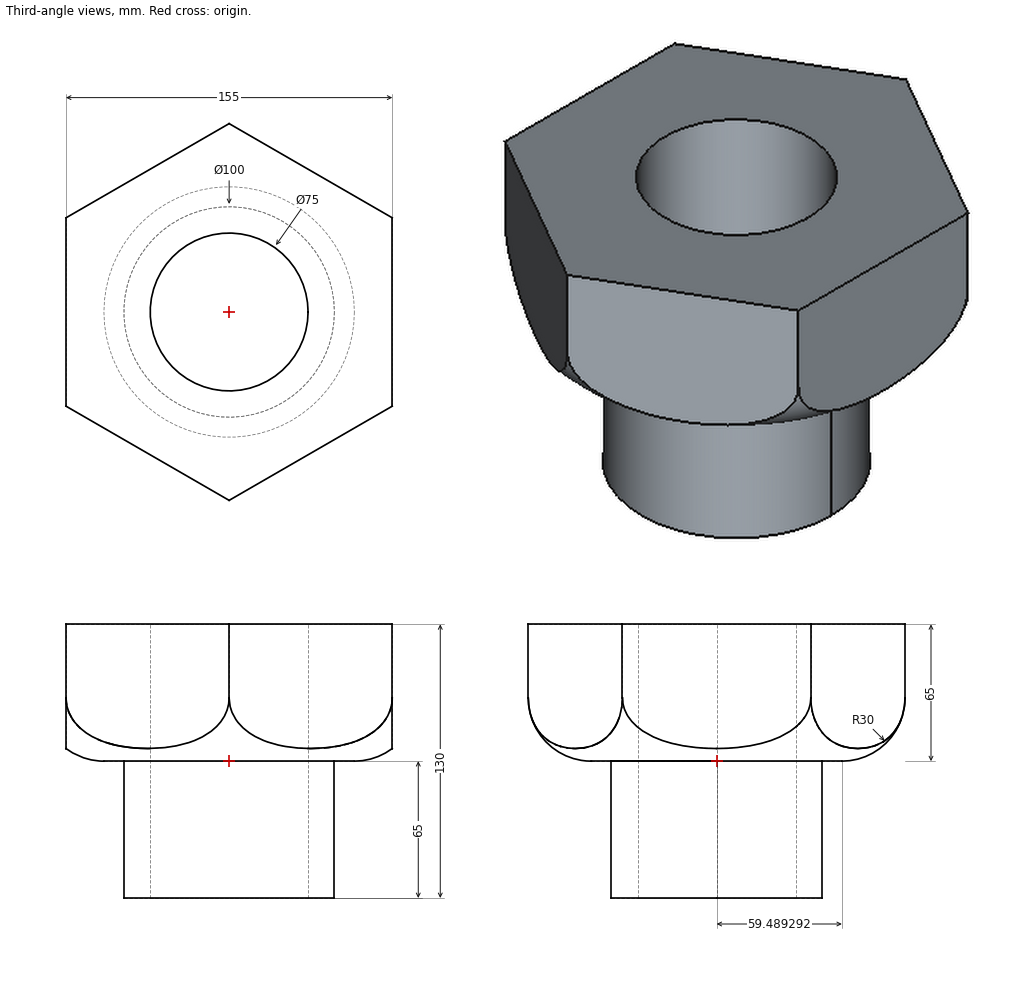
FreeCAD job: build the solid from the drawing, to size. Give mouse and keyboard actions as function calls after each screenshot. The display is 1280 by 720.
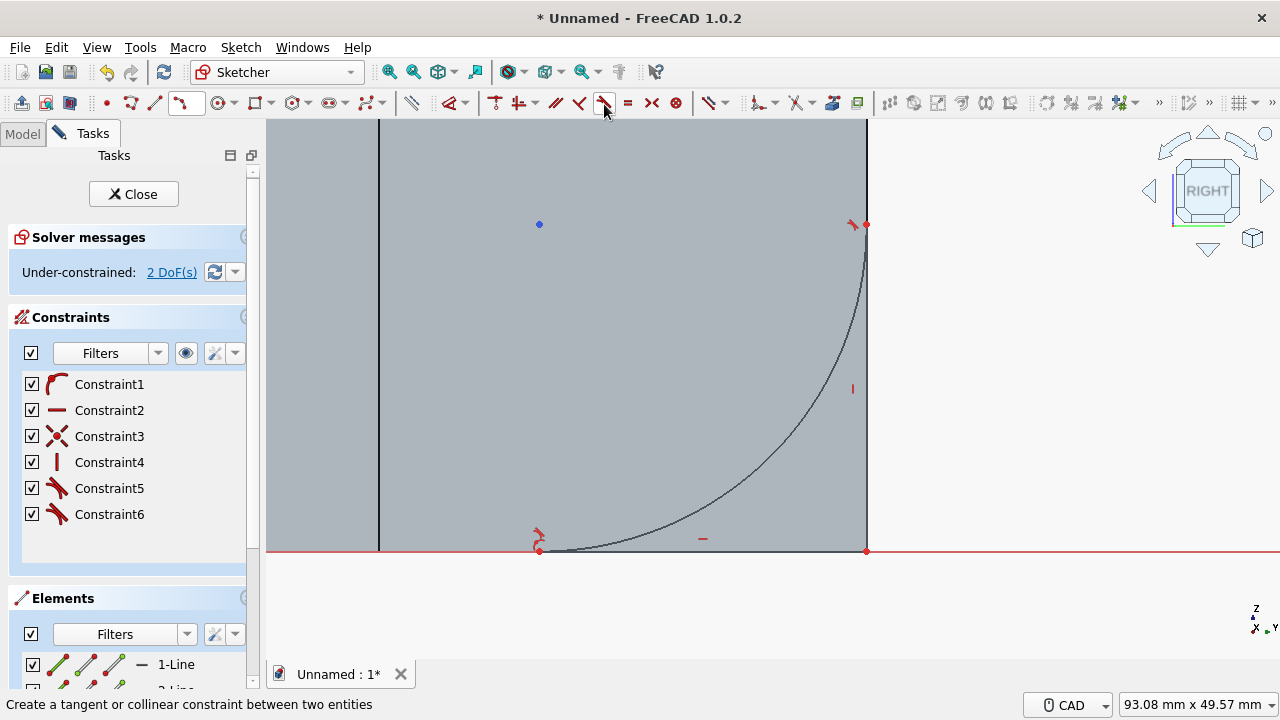
click(688, 516)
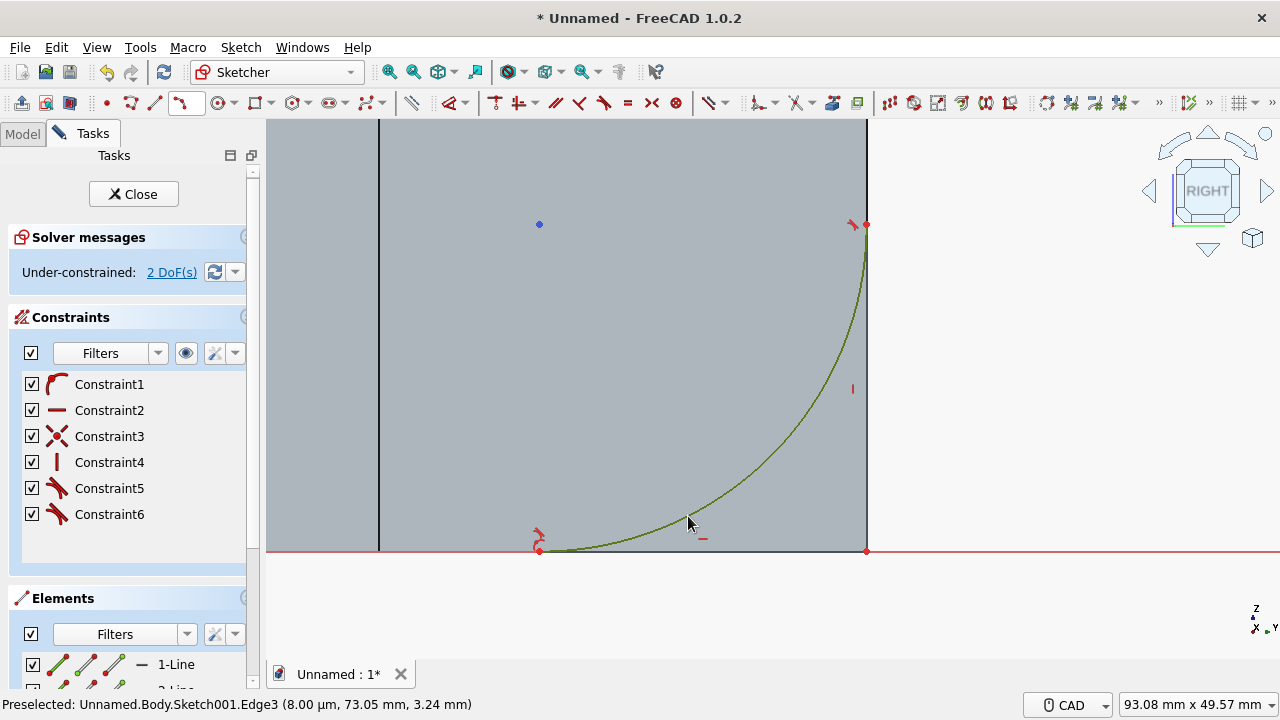
key(k)
key(r)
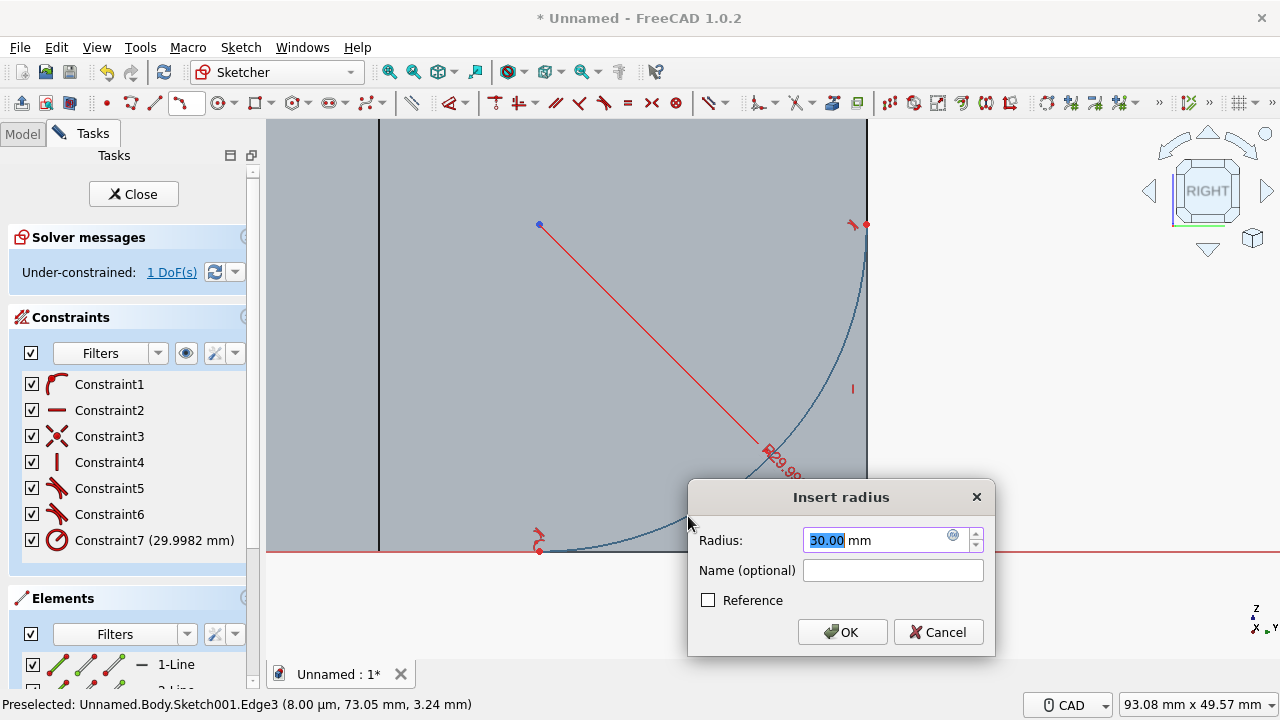
text(30)
key(Return)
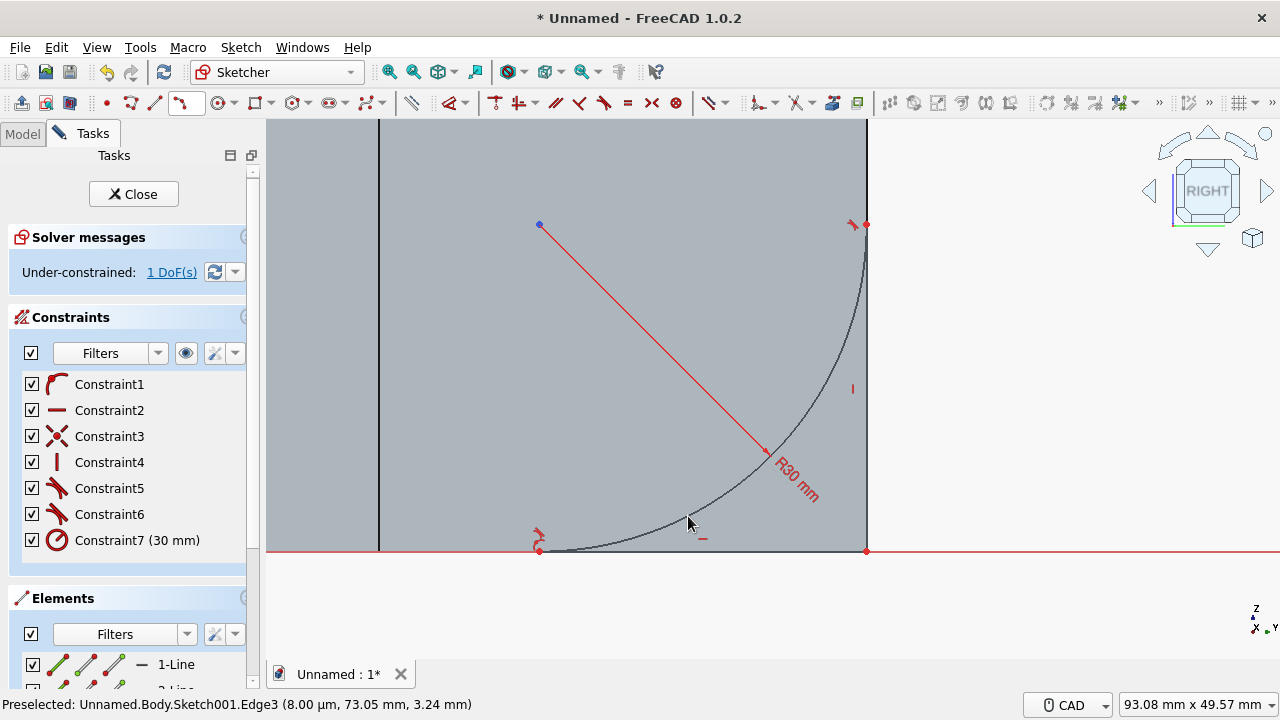
click(540, 552)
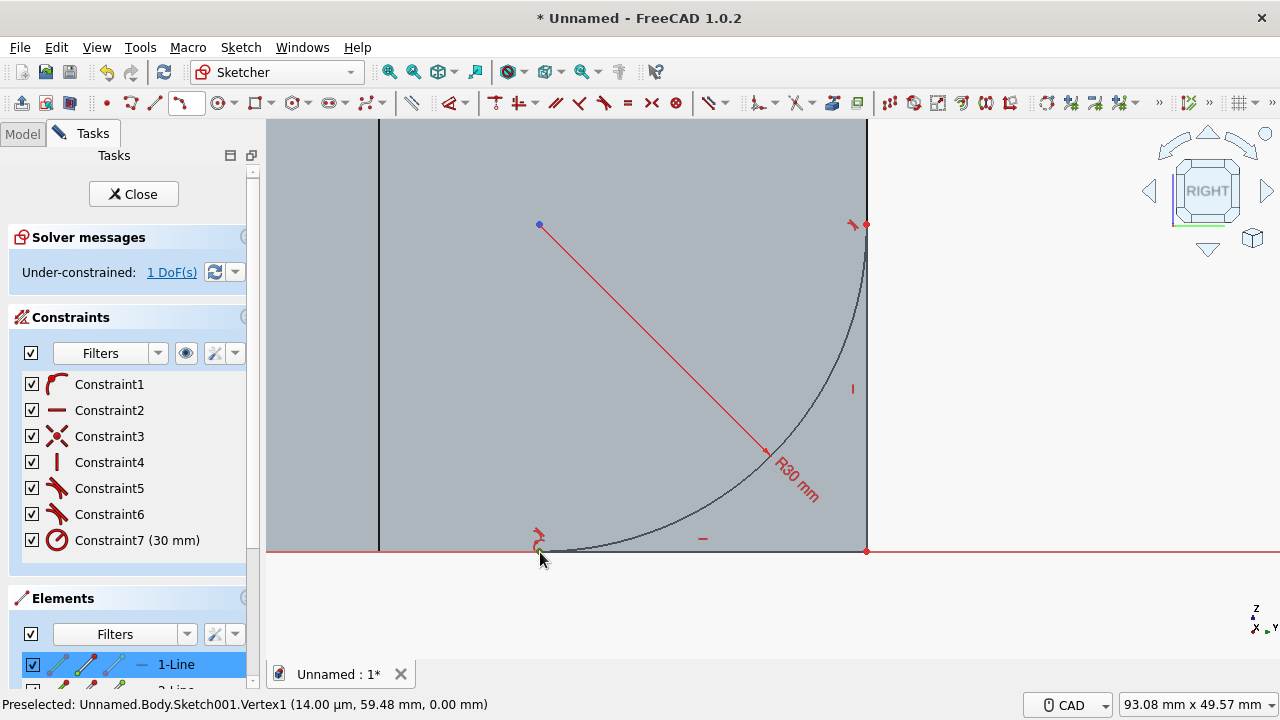
key(l)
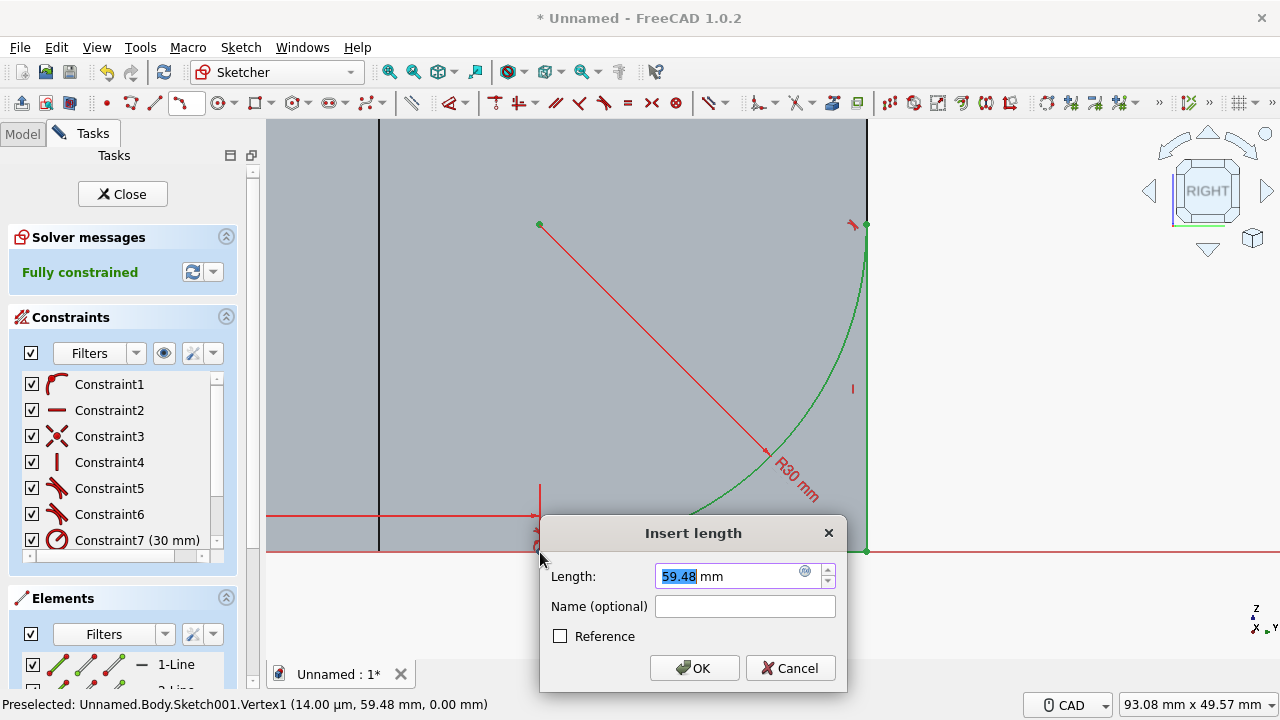
text(59.489292)
key(Return)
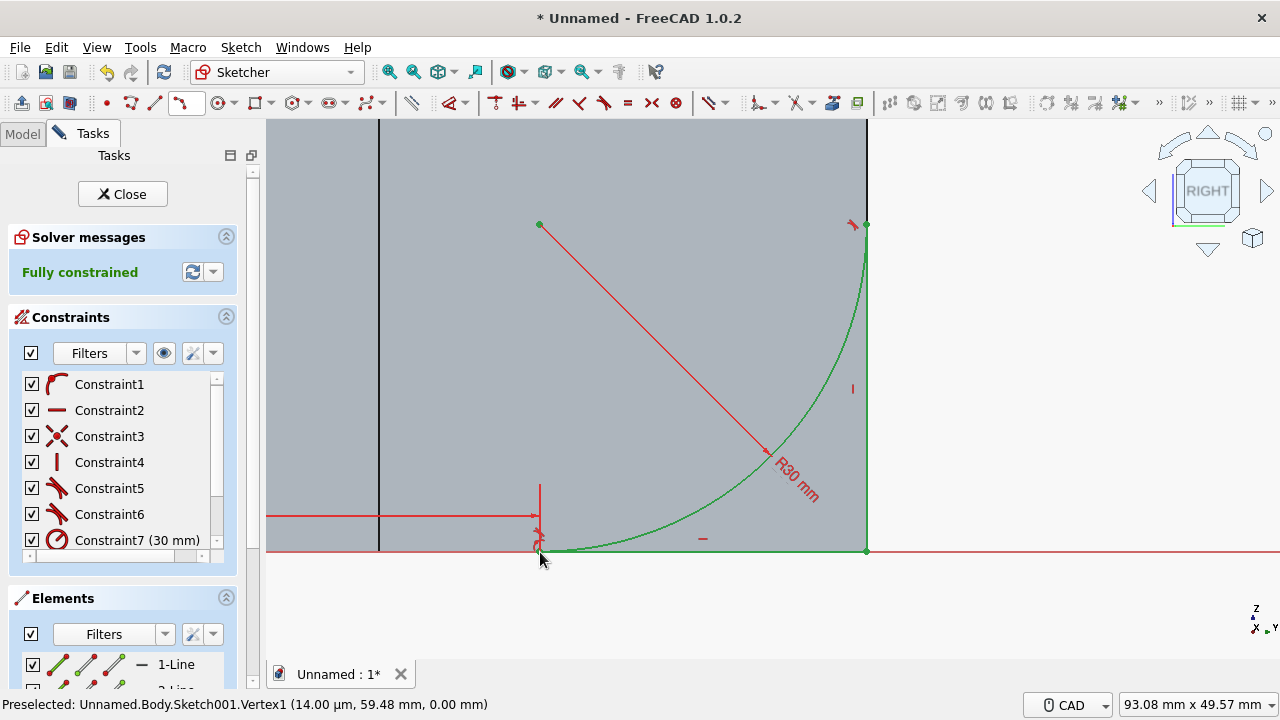
click(123, 194)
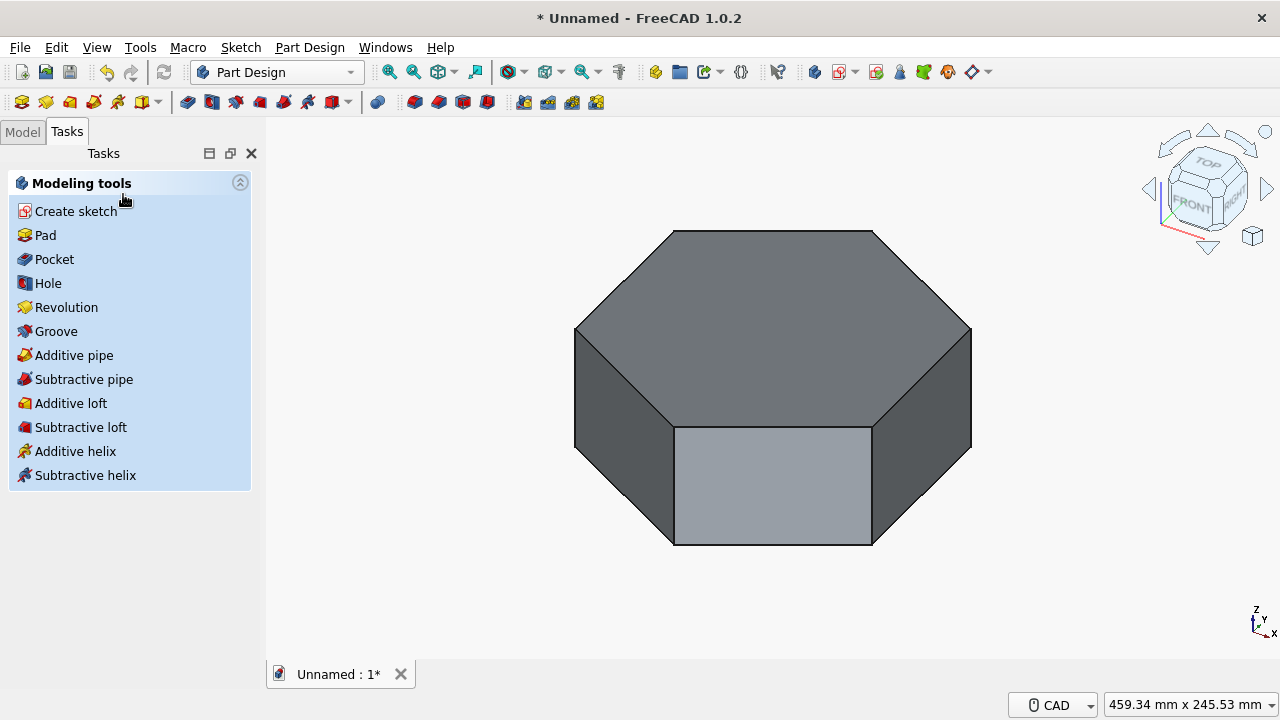
click(236, 102)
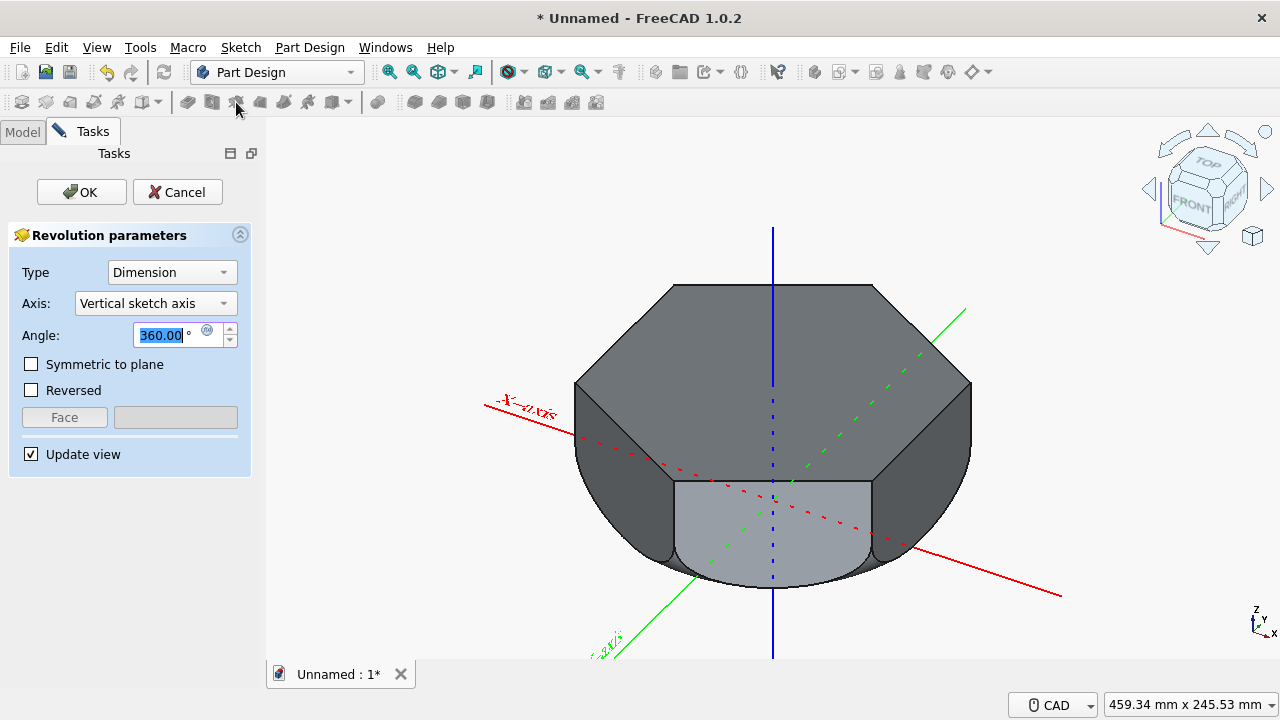
click(82, 192)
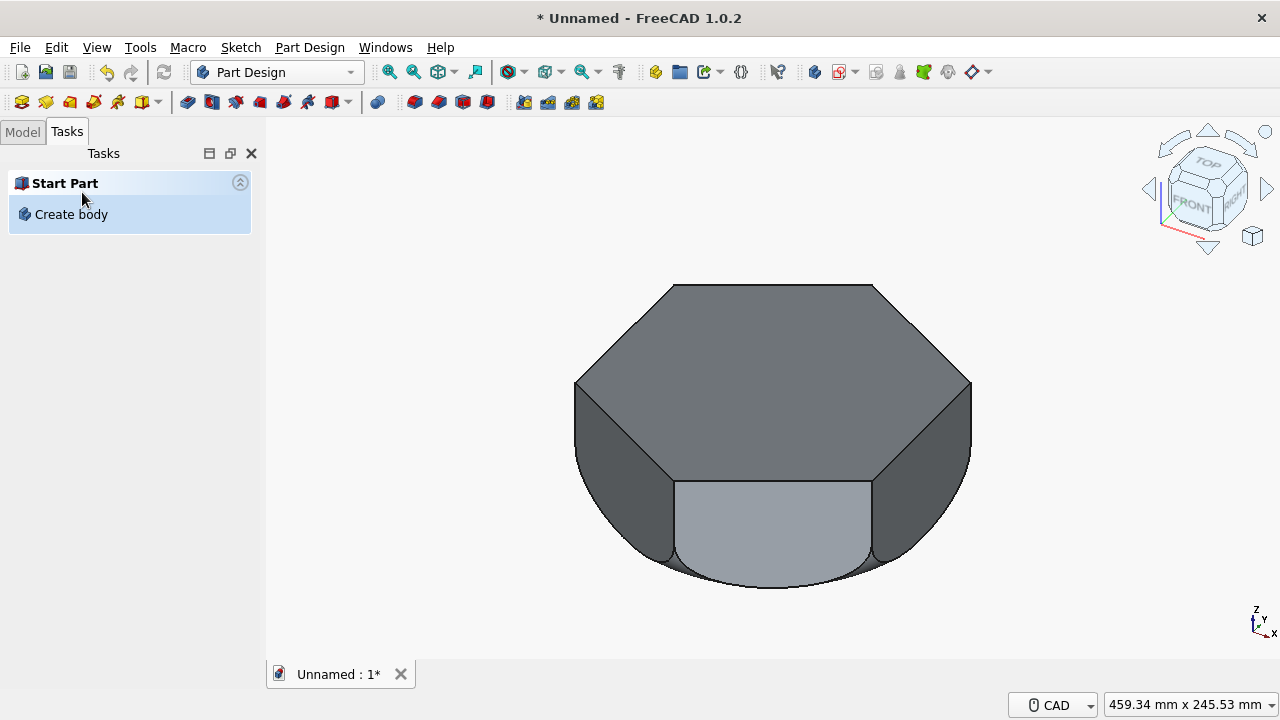
key(5)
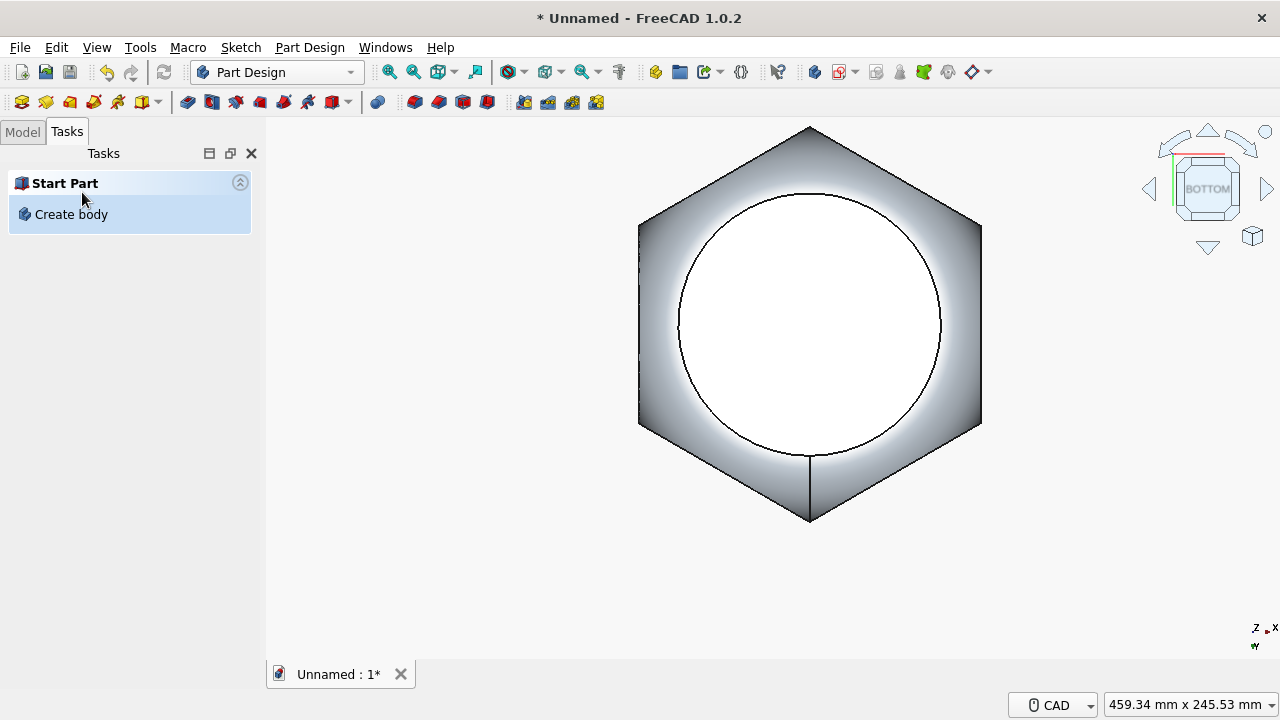
click(810, 324)